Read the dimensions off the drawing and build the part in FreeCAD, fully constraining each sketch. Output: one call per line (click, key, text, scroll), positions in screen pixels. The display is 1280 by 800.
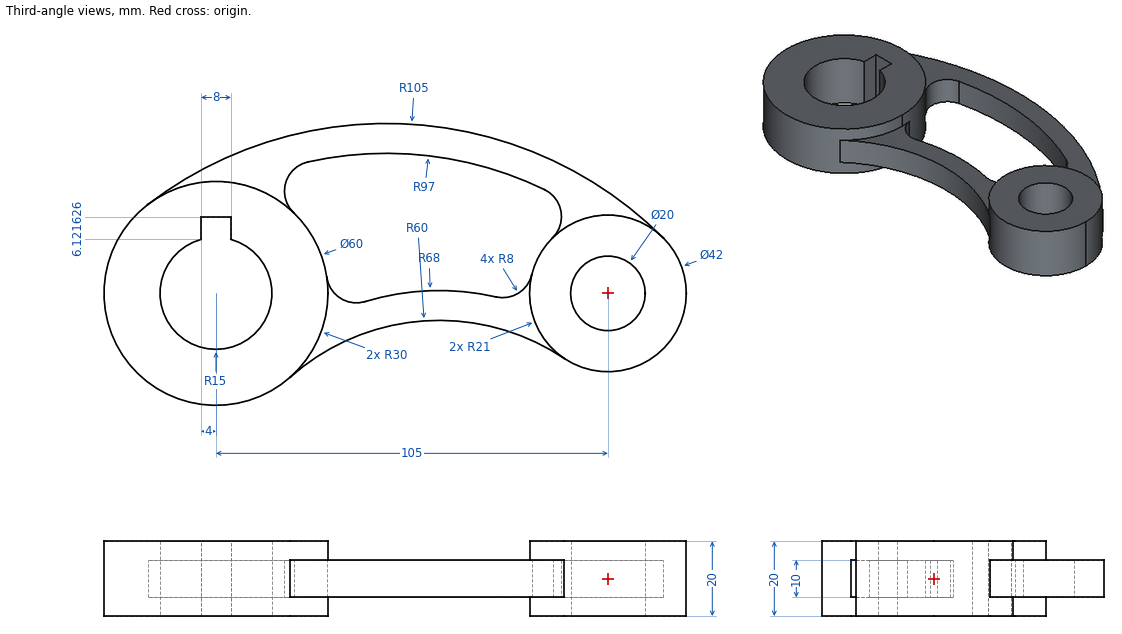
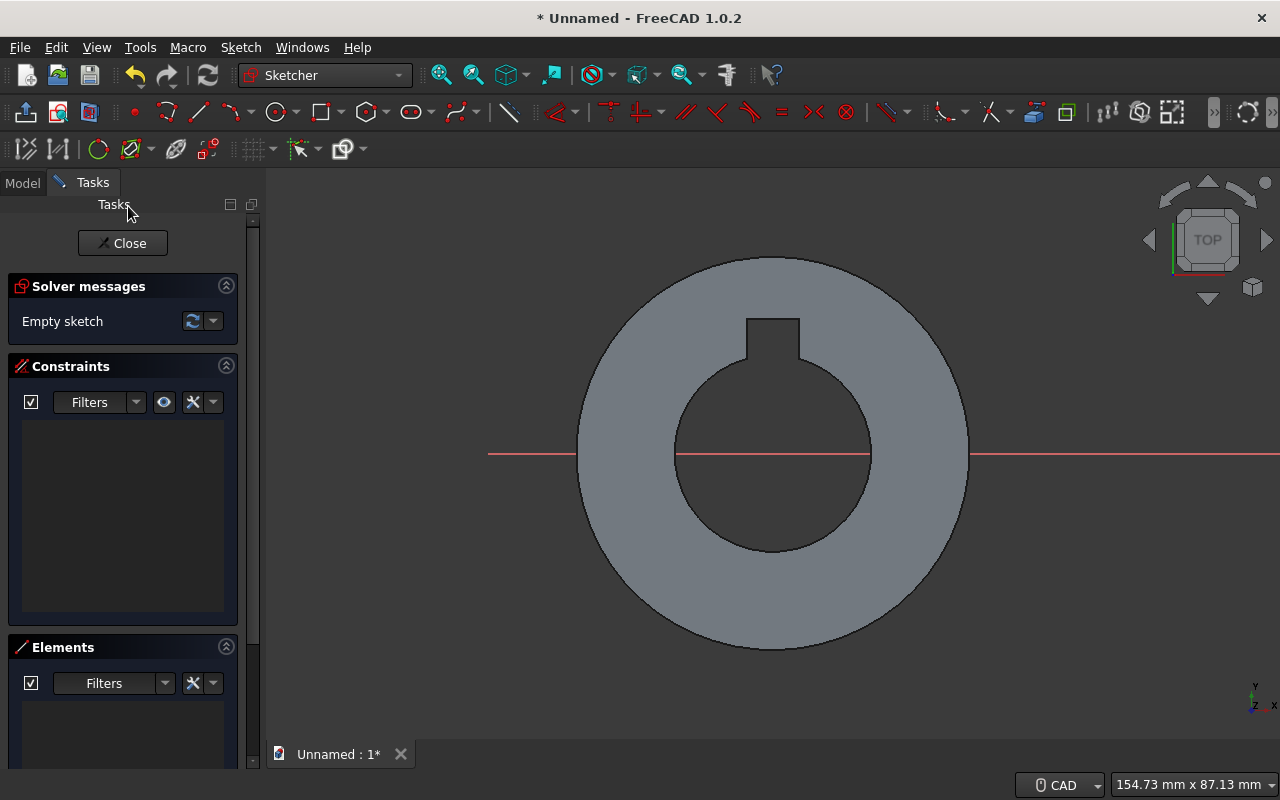
scroll(704, 454, down, 5)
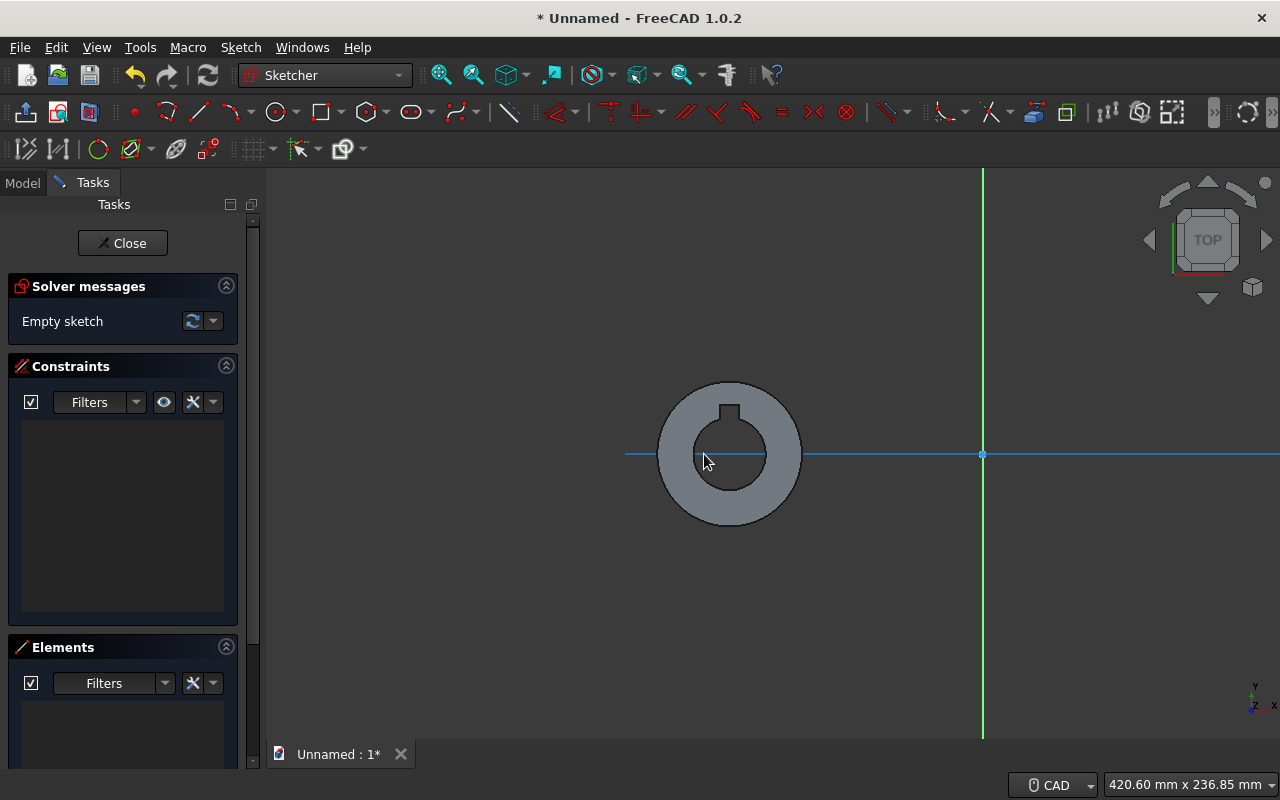
scroll(1103, 454, up, 6)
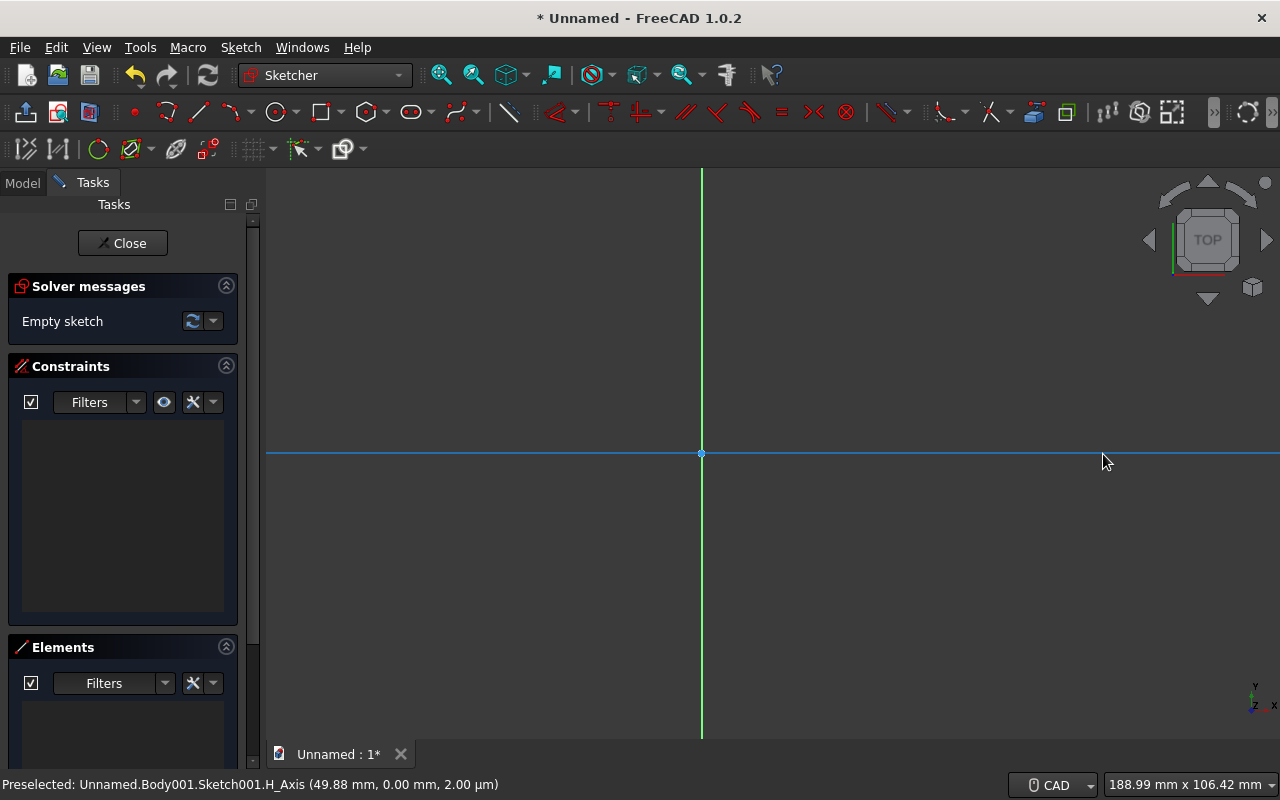
key(g)
key(c)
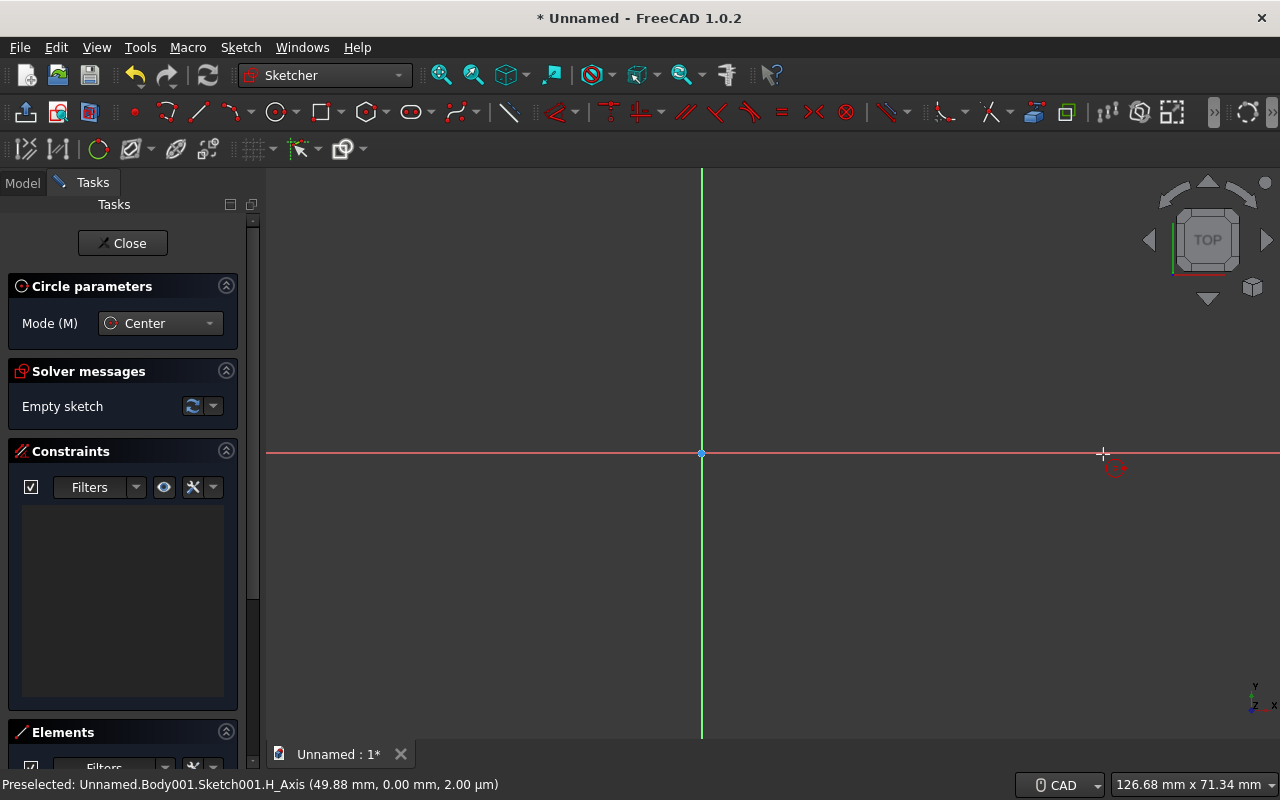
click(702, 453)
move(821, 334)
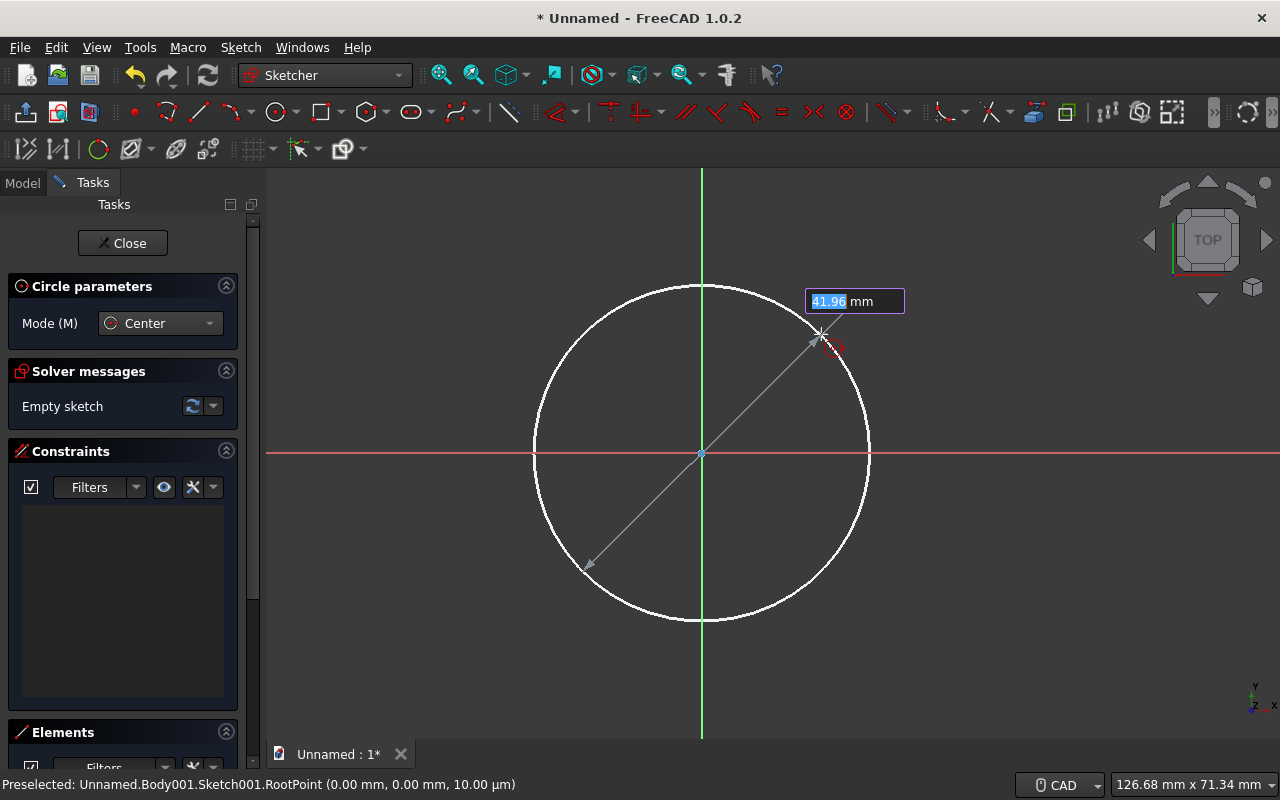
text(42)
key(Return)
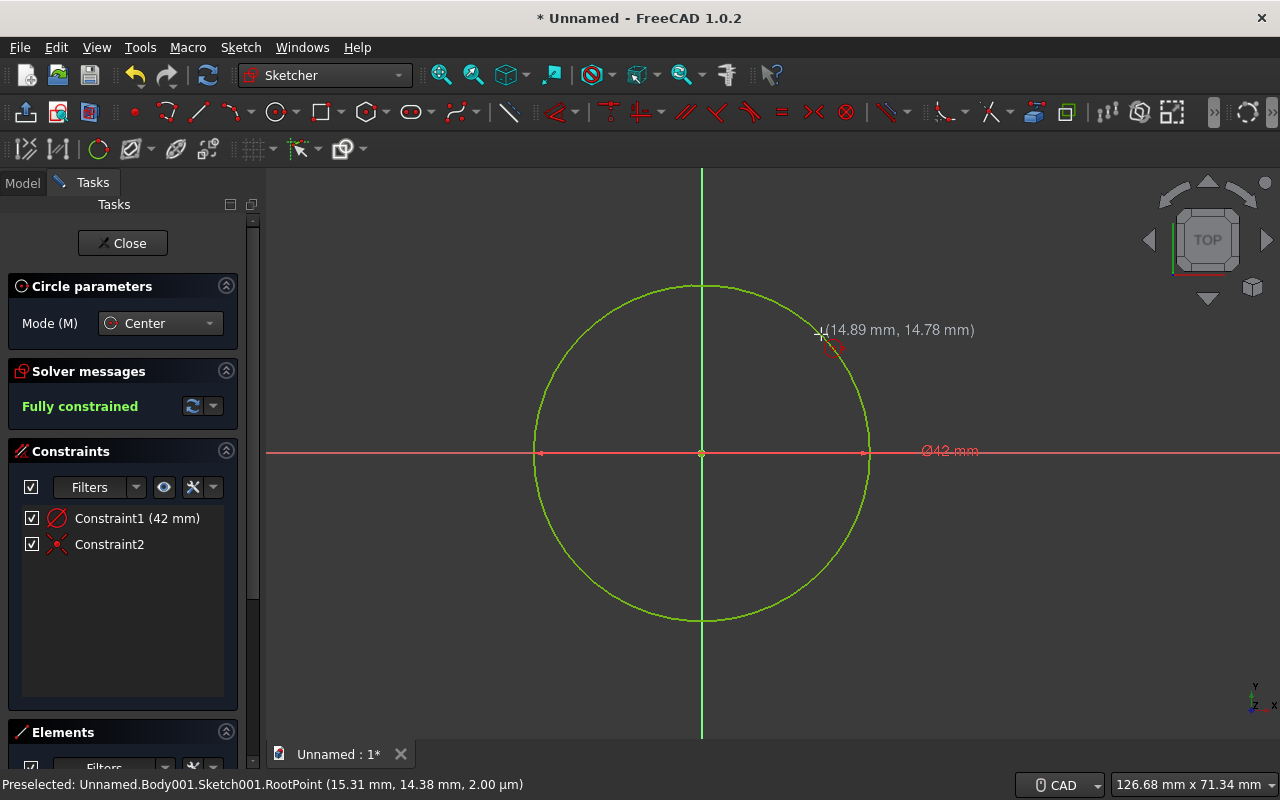
click(702, 453)
move(758, 397)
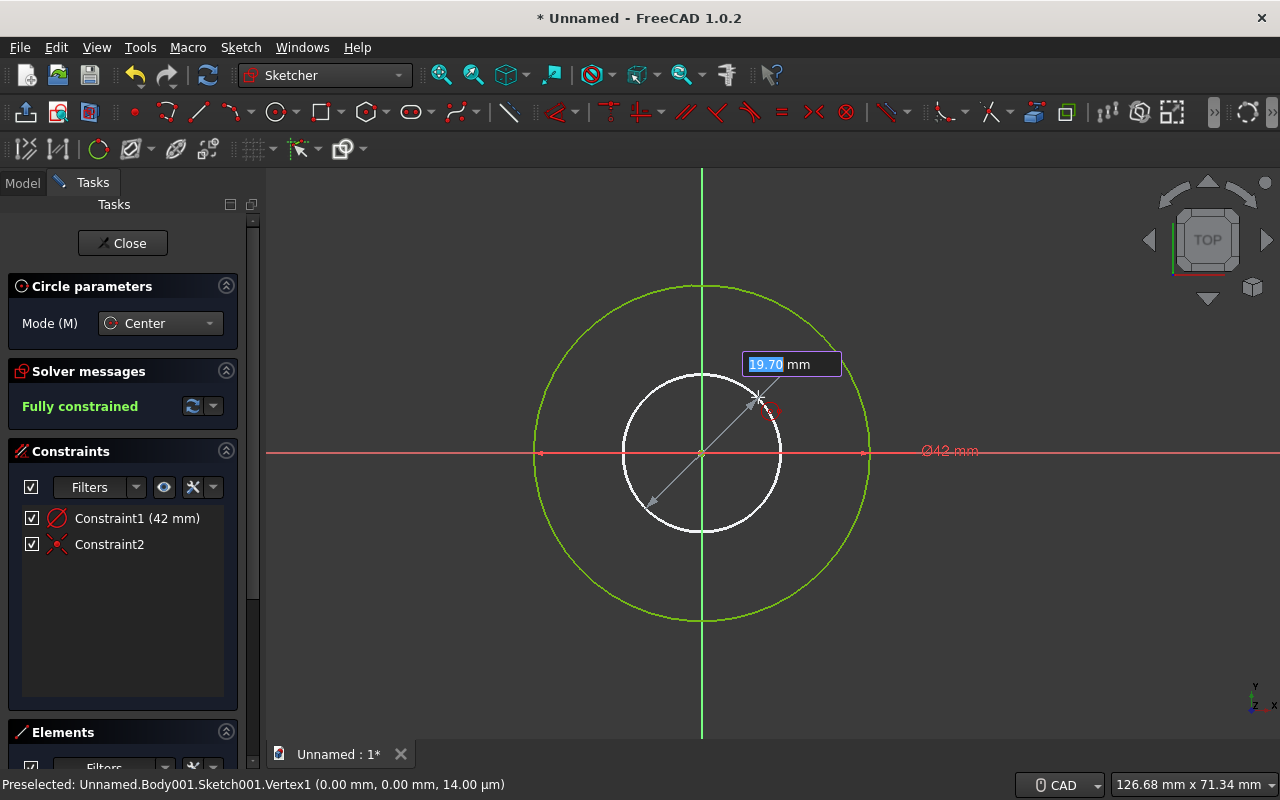
text(20)
key(Return)
key(Escape)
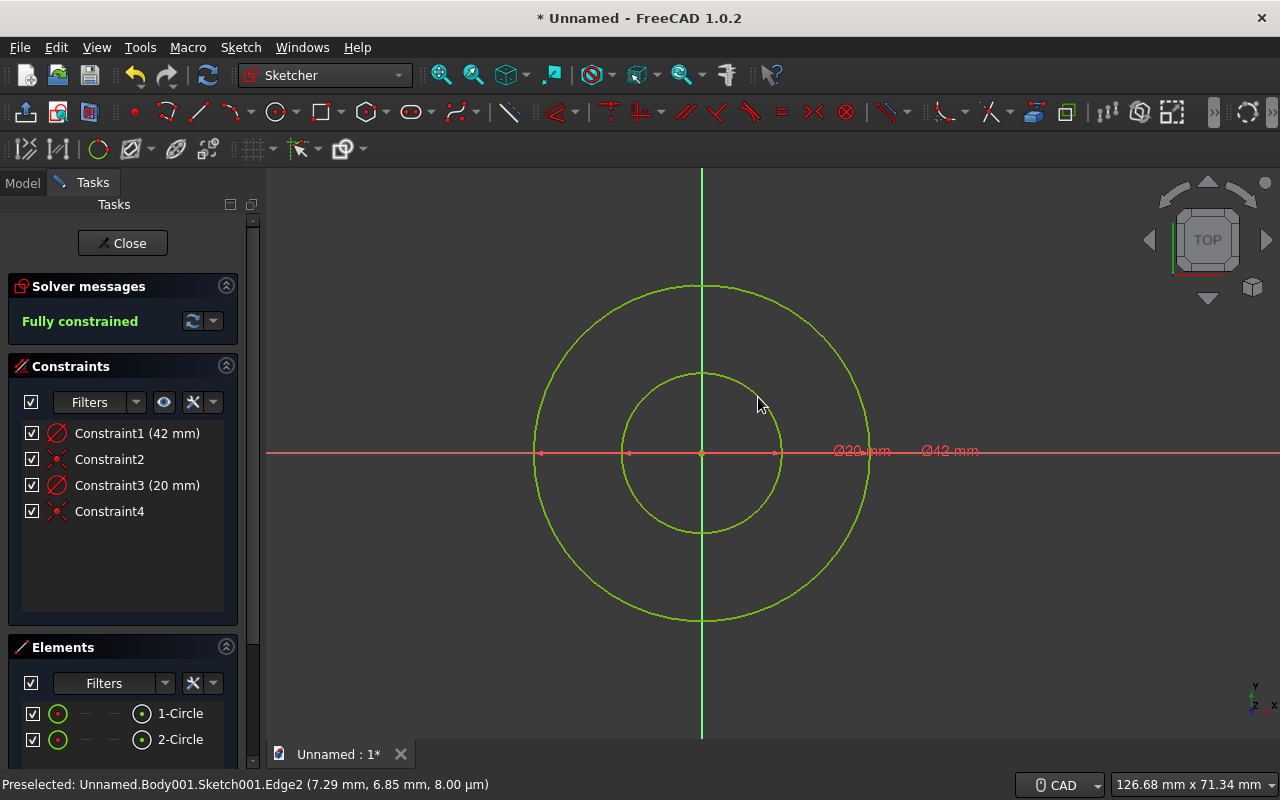
click(123, 243)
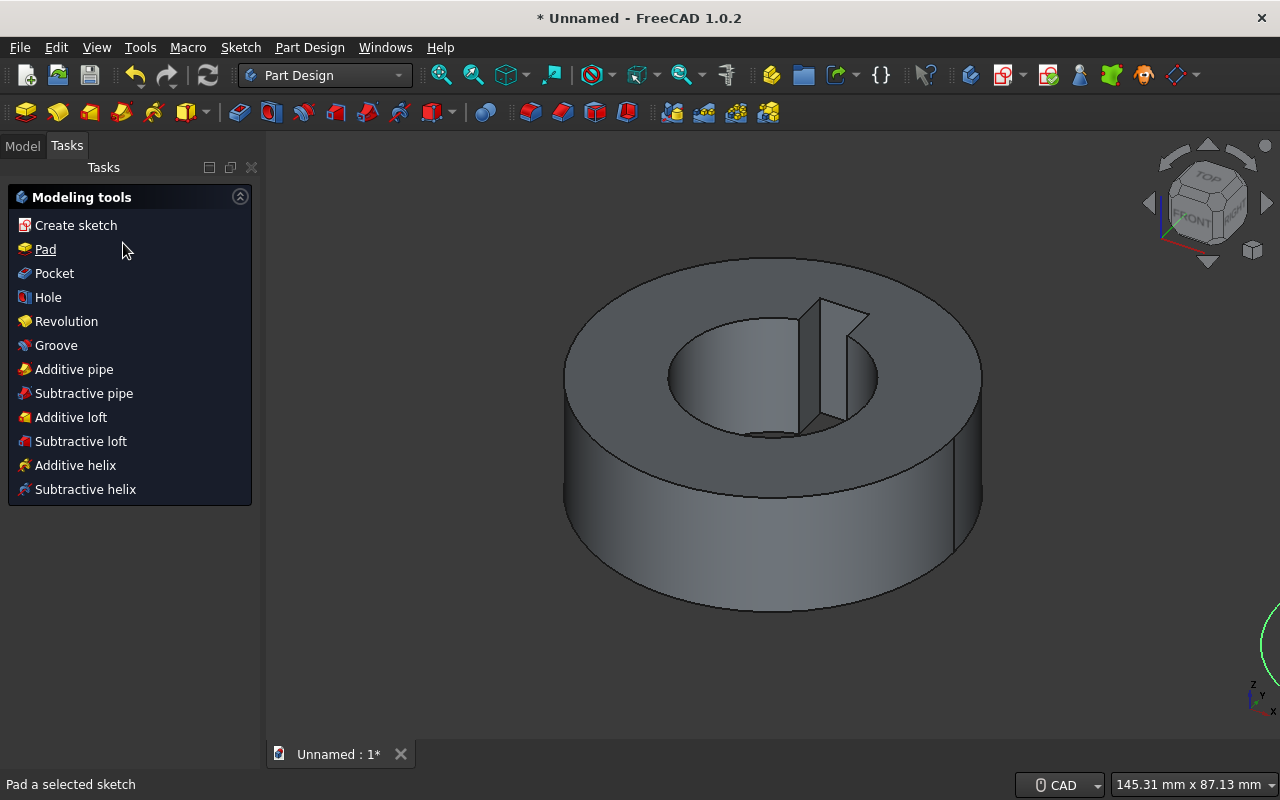
click(26, 112)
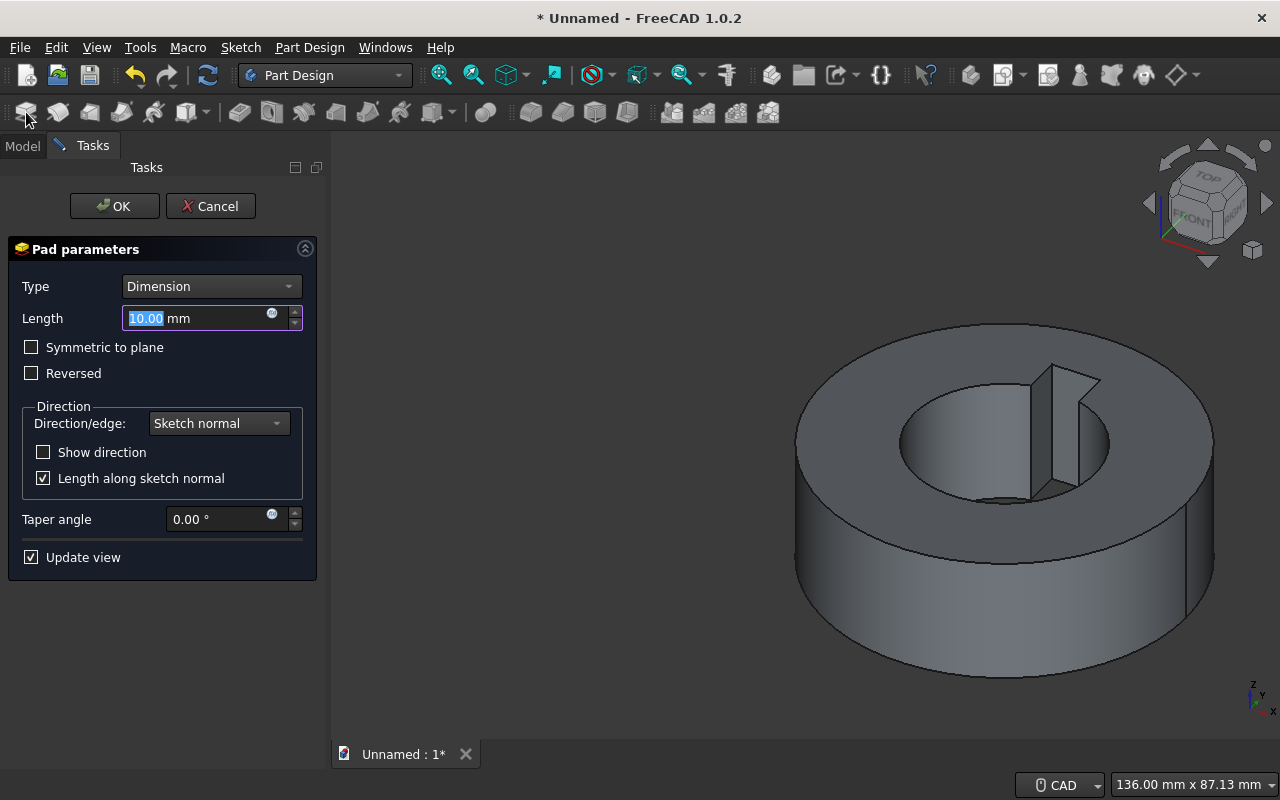
text(20)
key(Tab)